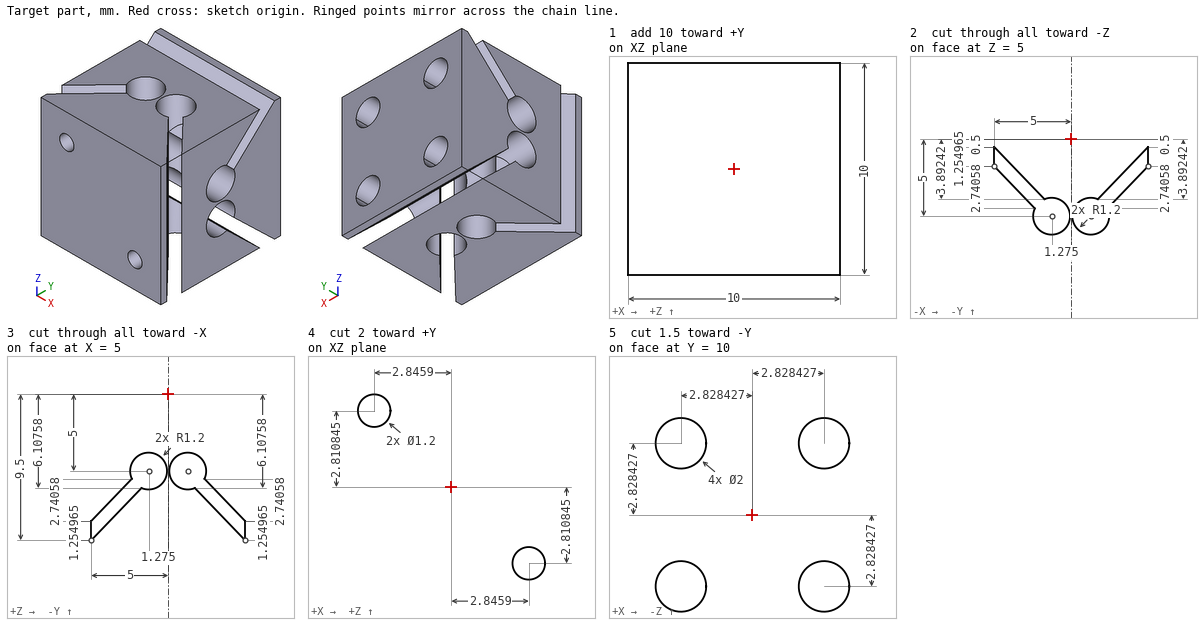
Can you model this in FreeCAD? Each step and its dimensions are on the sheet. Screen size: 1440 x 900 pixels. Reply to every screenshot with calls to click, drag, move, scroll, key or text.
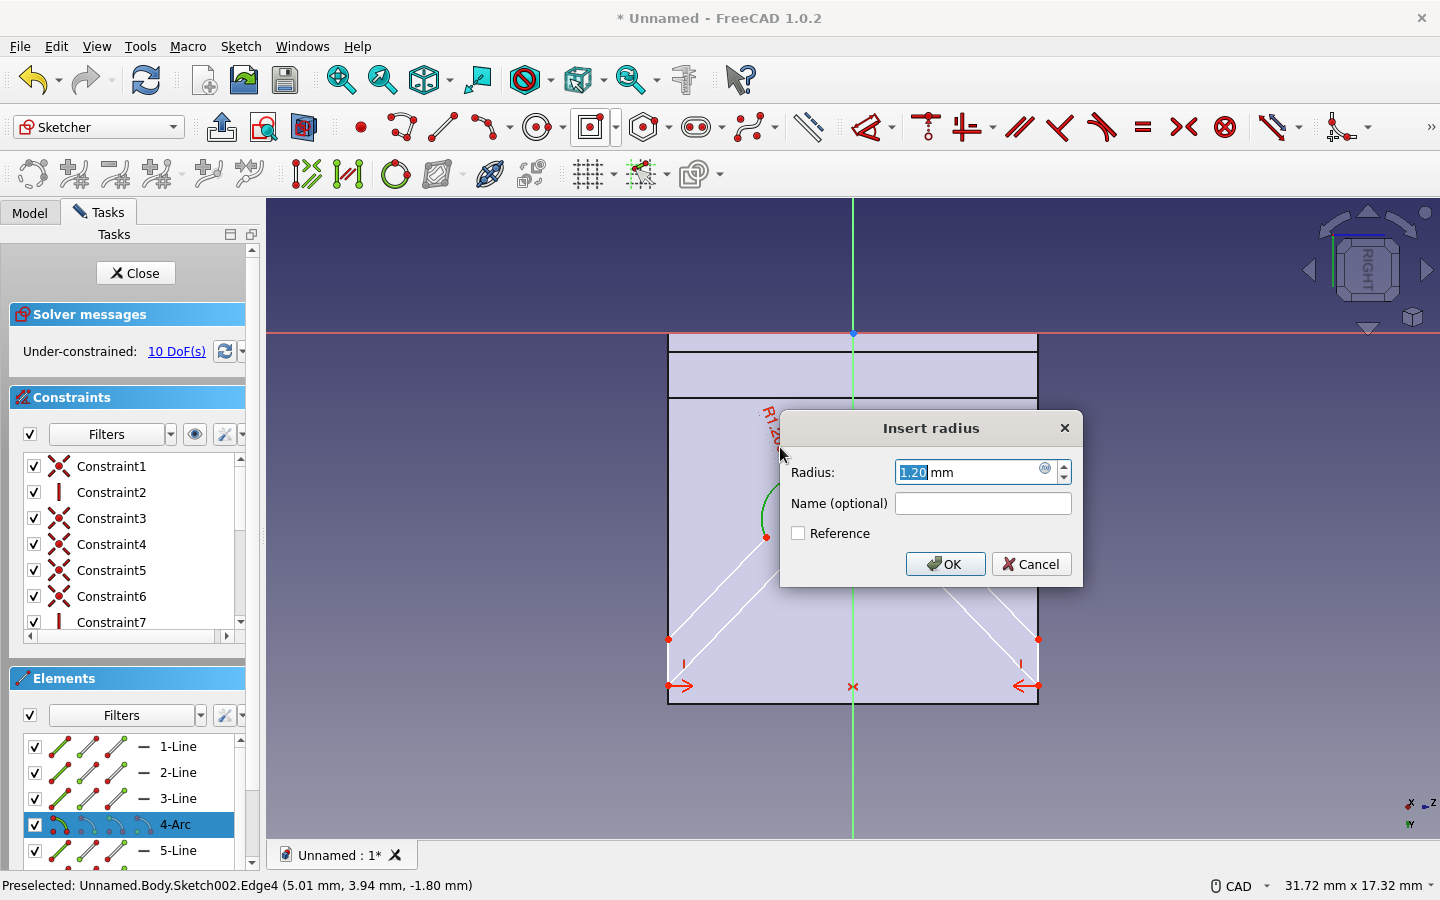
text(1.2)
key(Return)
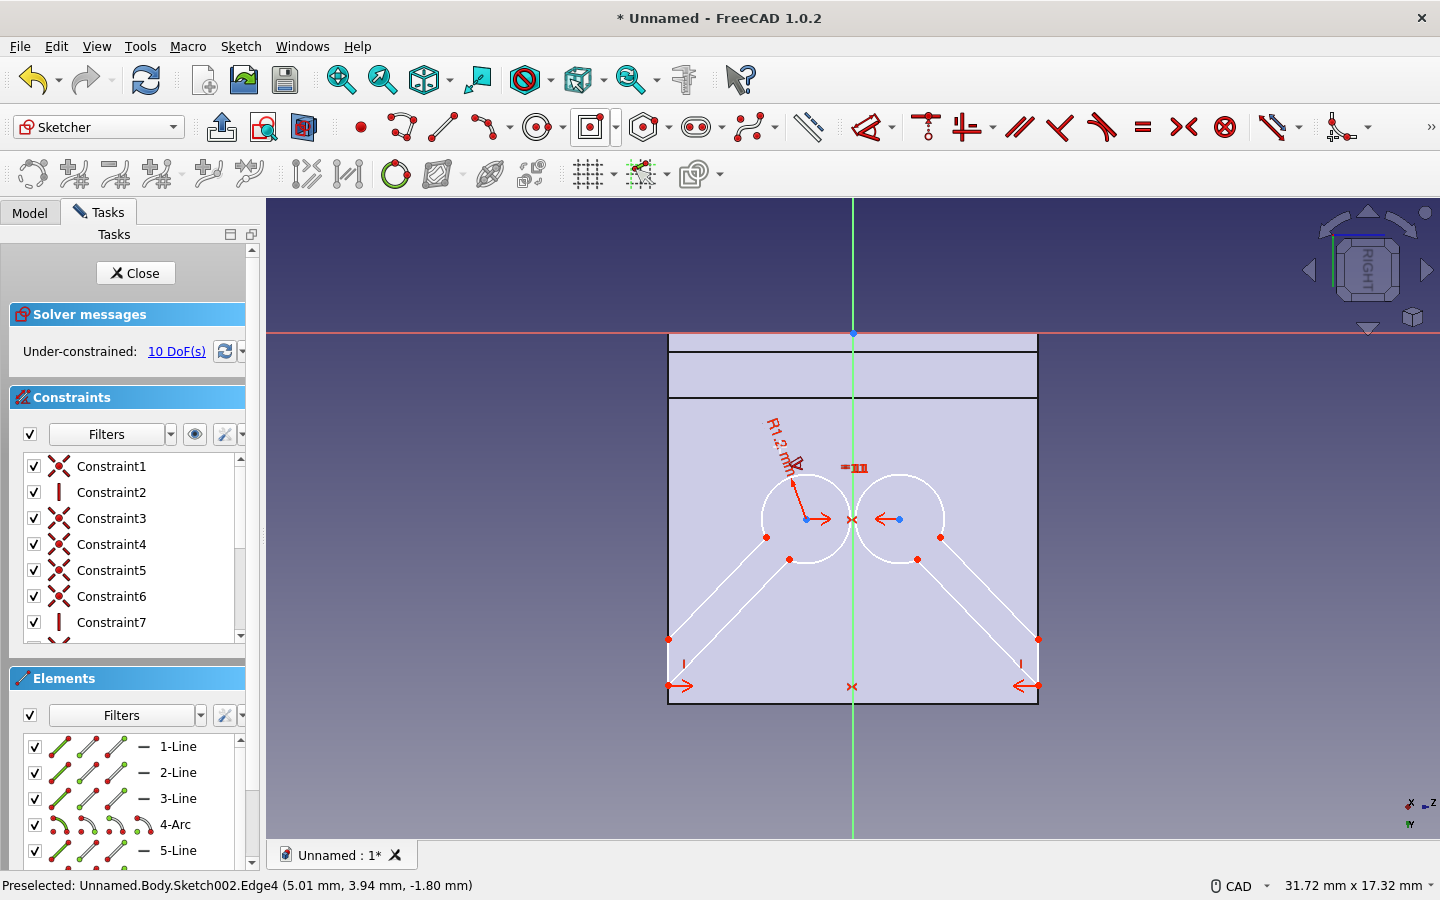
click(668, 640)
click(760, 299)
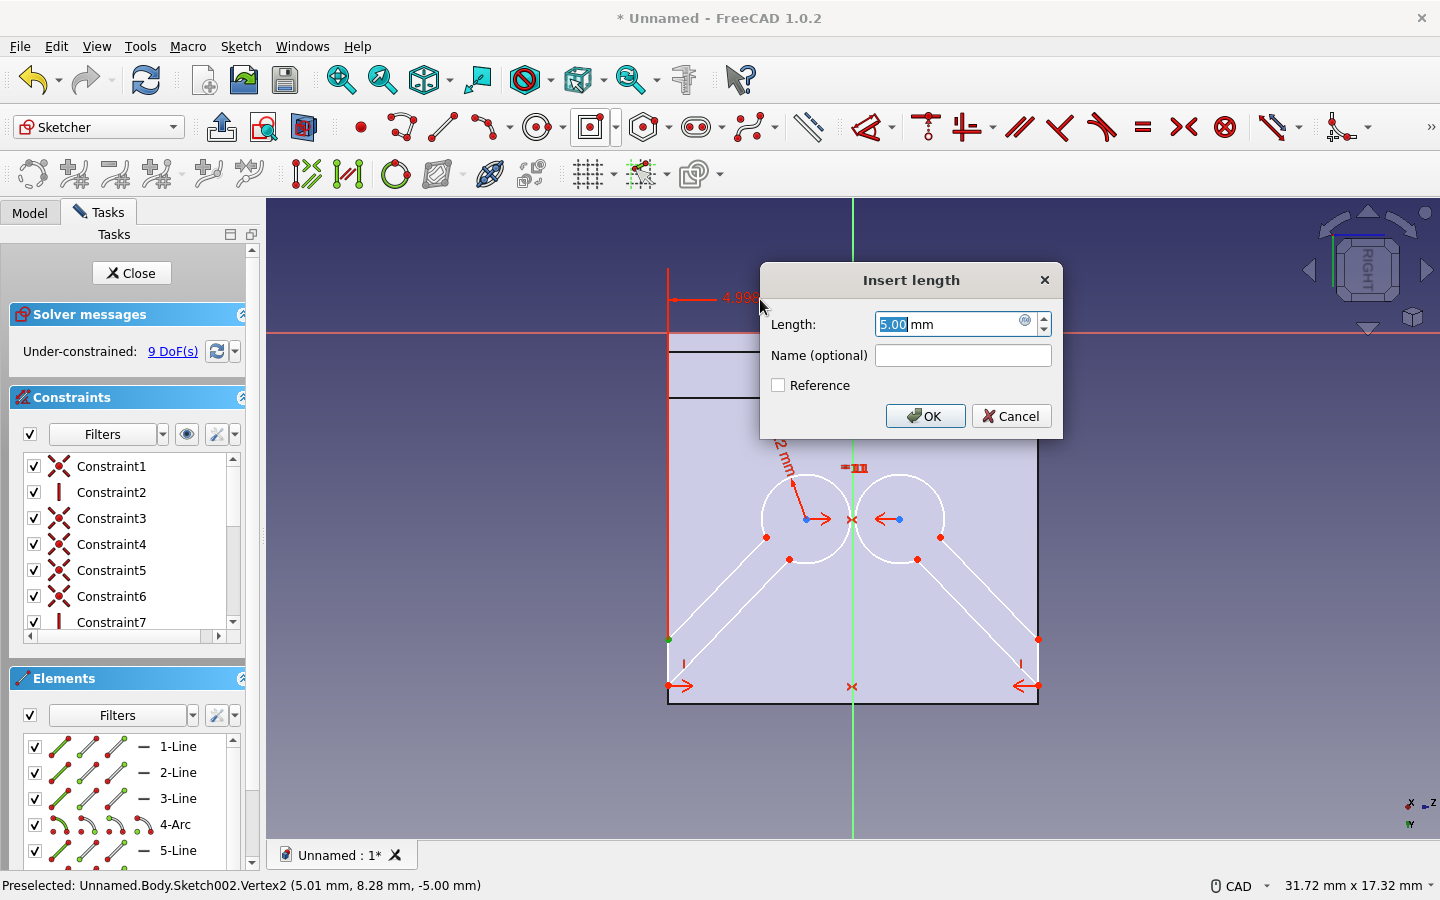
text(5)
key(Return)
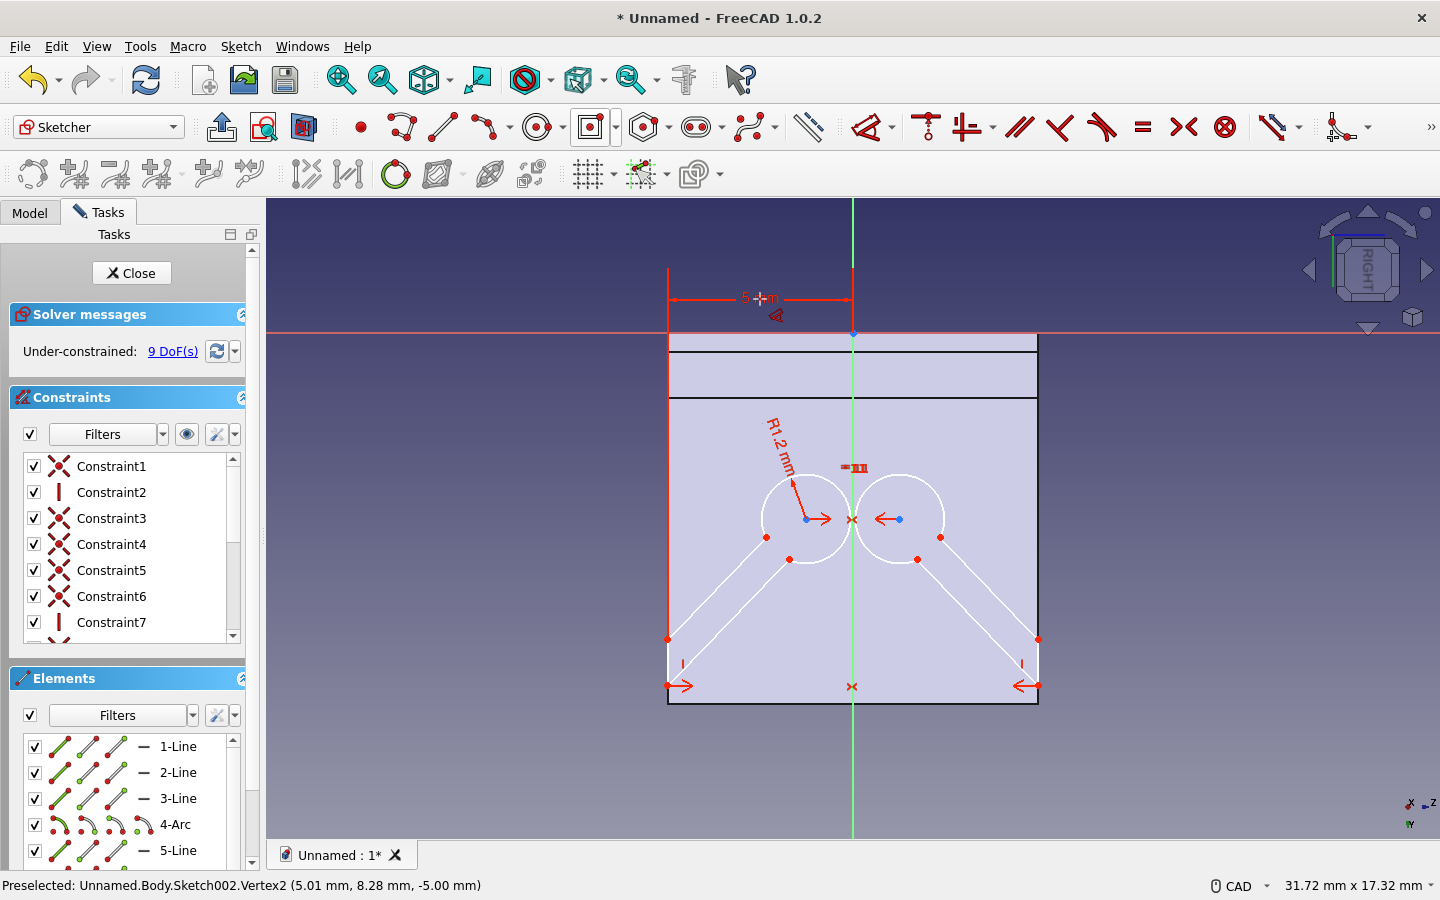
click(806, 519)
click(772, 426)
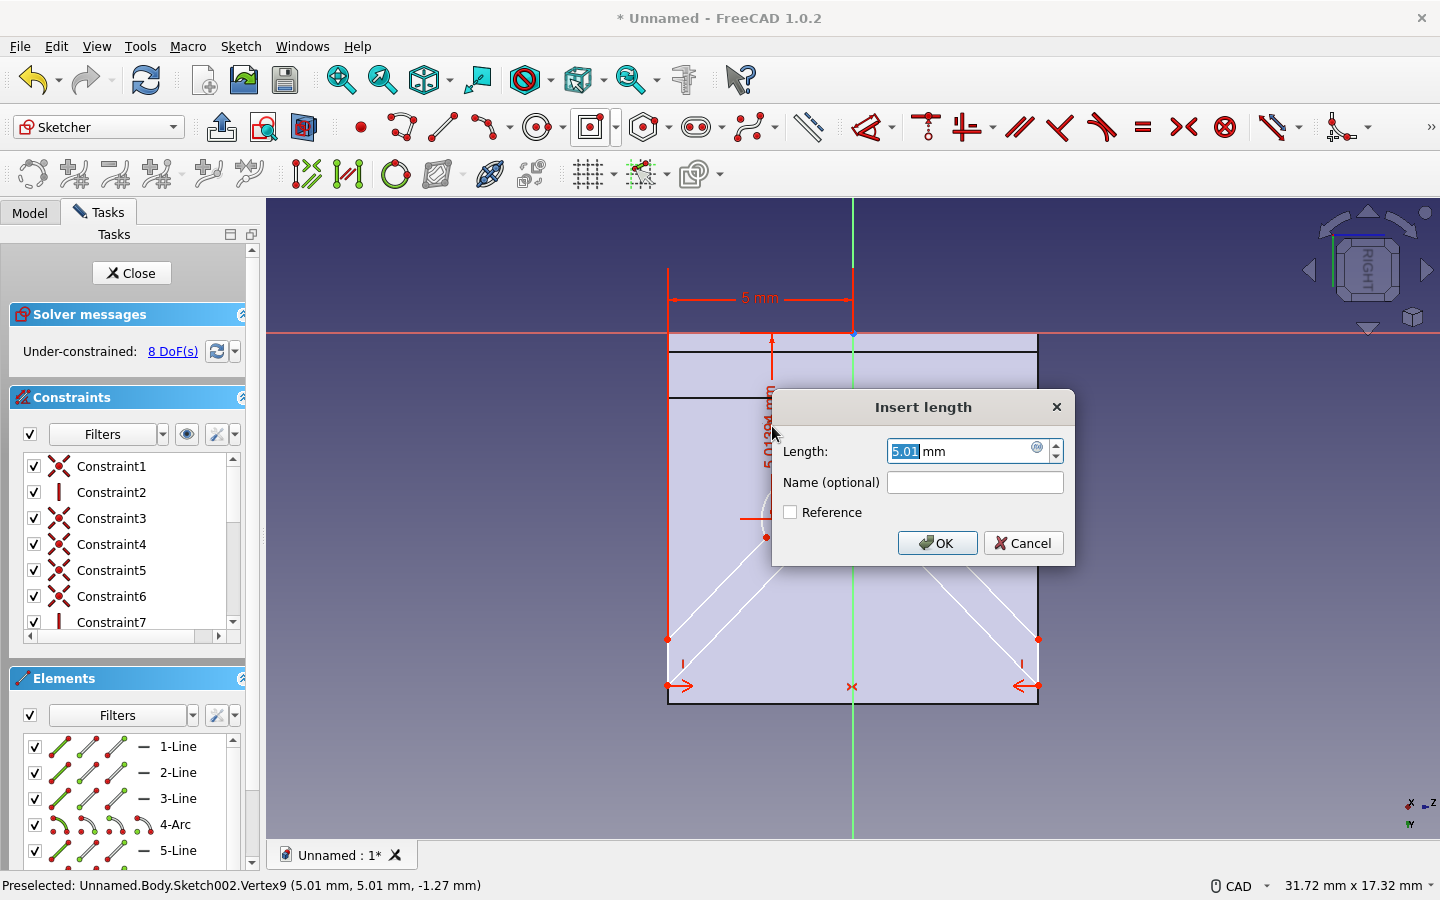
text(5)
key(Return)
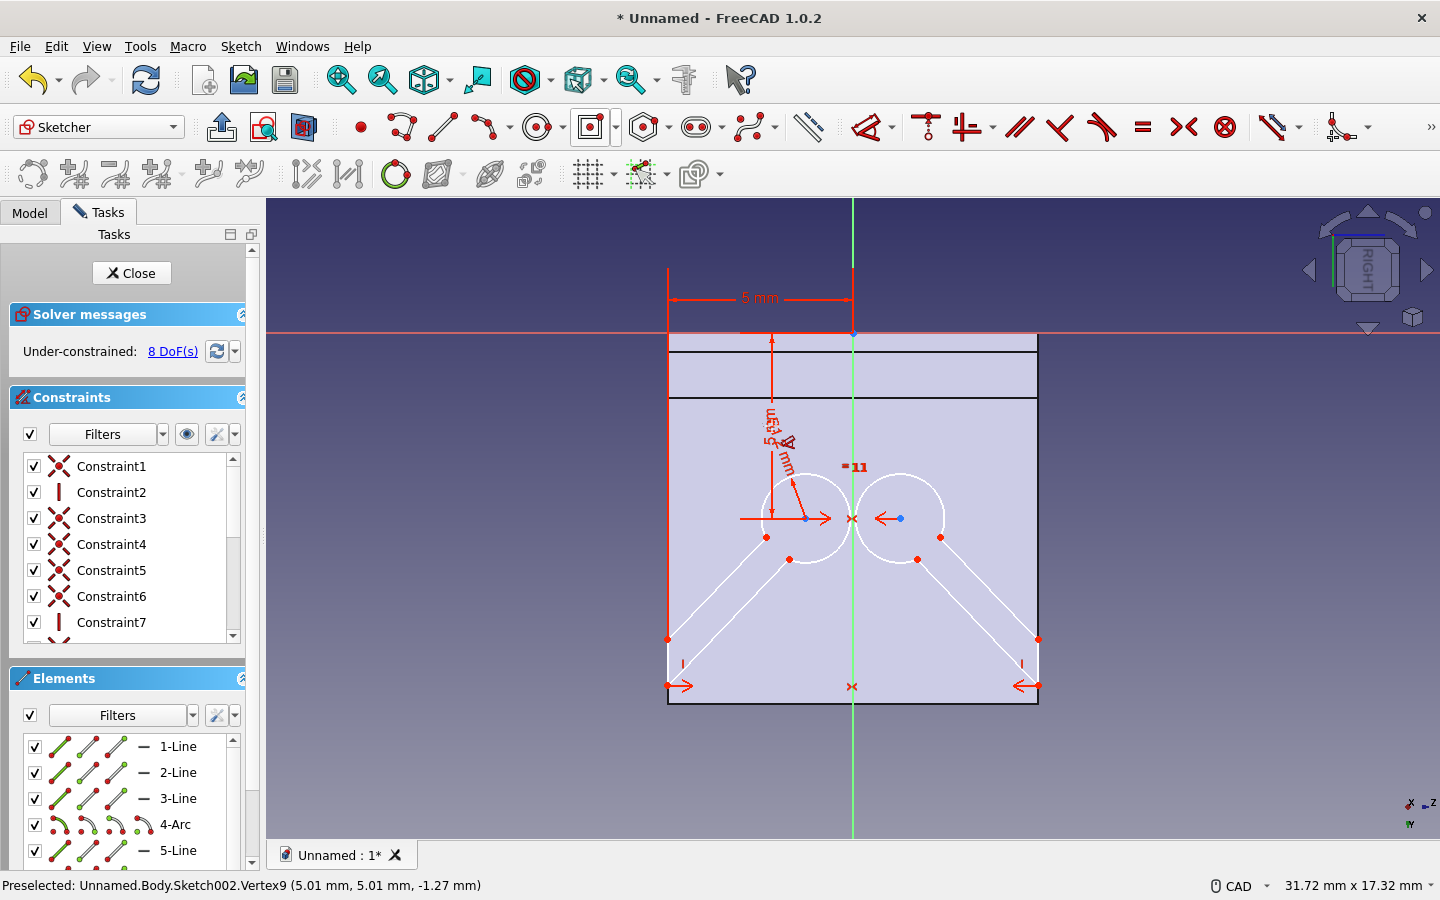
click(668, 686)
click(634, 510)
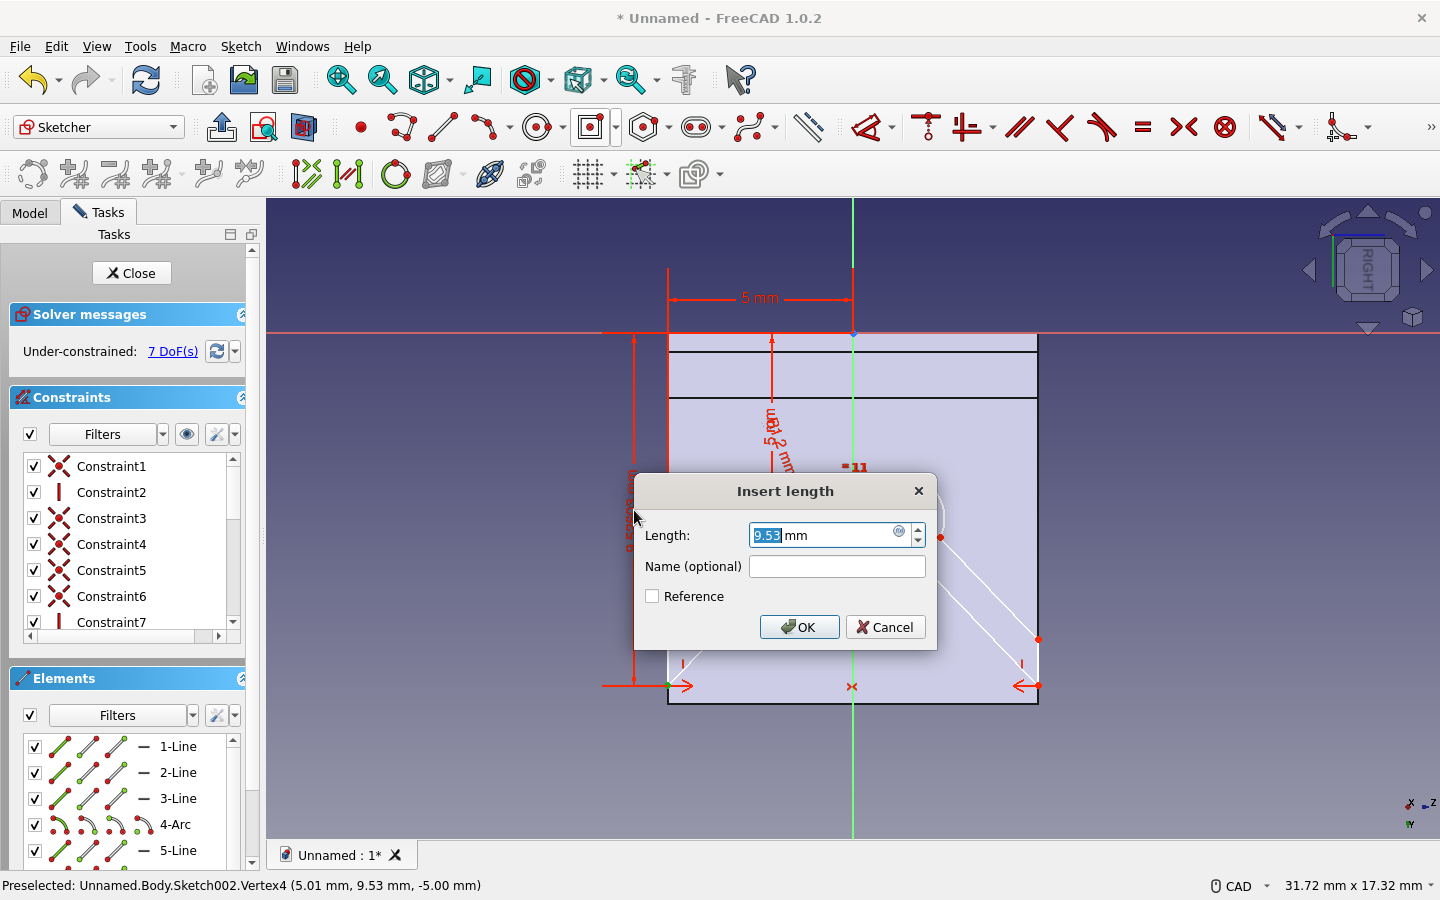
text(9.5)
key(Return)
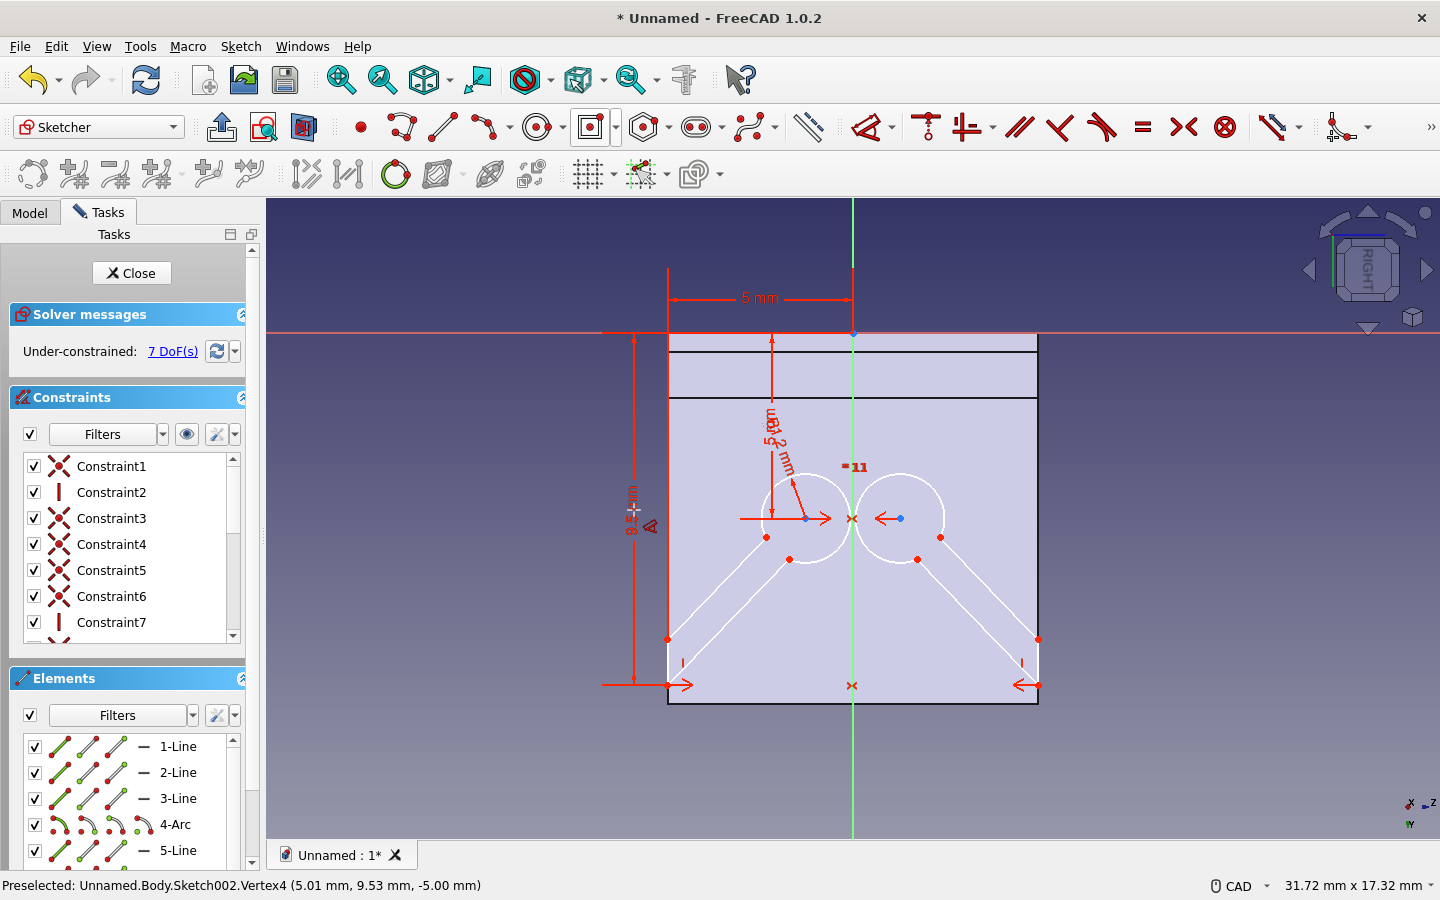
click(806, 518)
click(829, 275)